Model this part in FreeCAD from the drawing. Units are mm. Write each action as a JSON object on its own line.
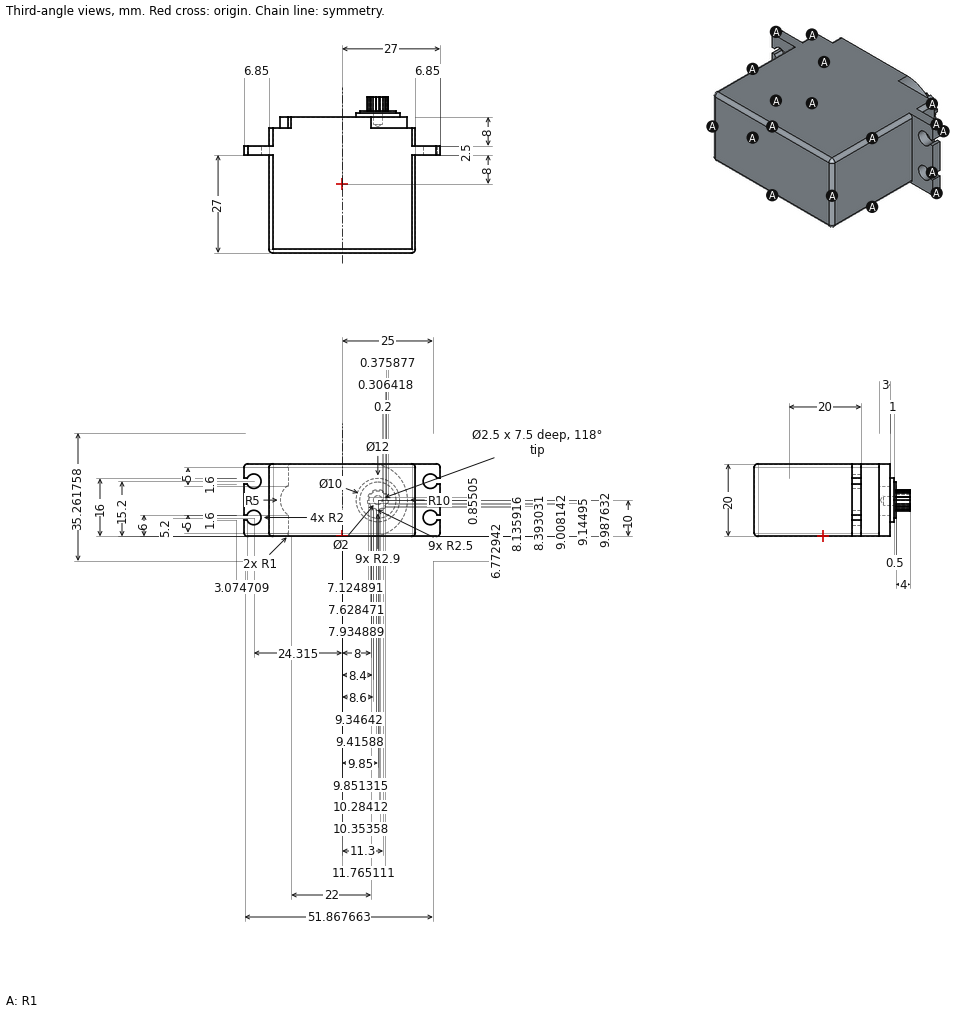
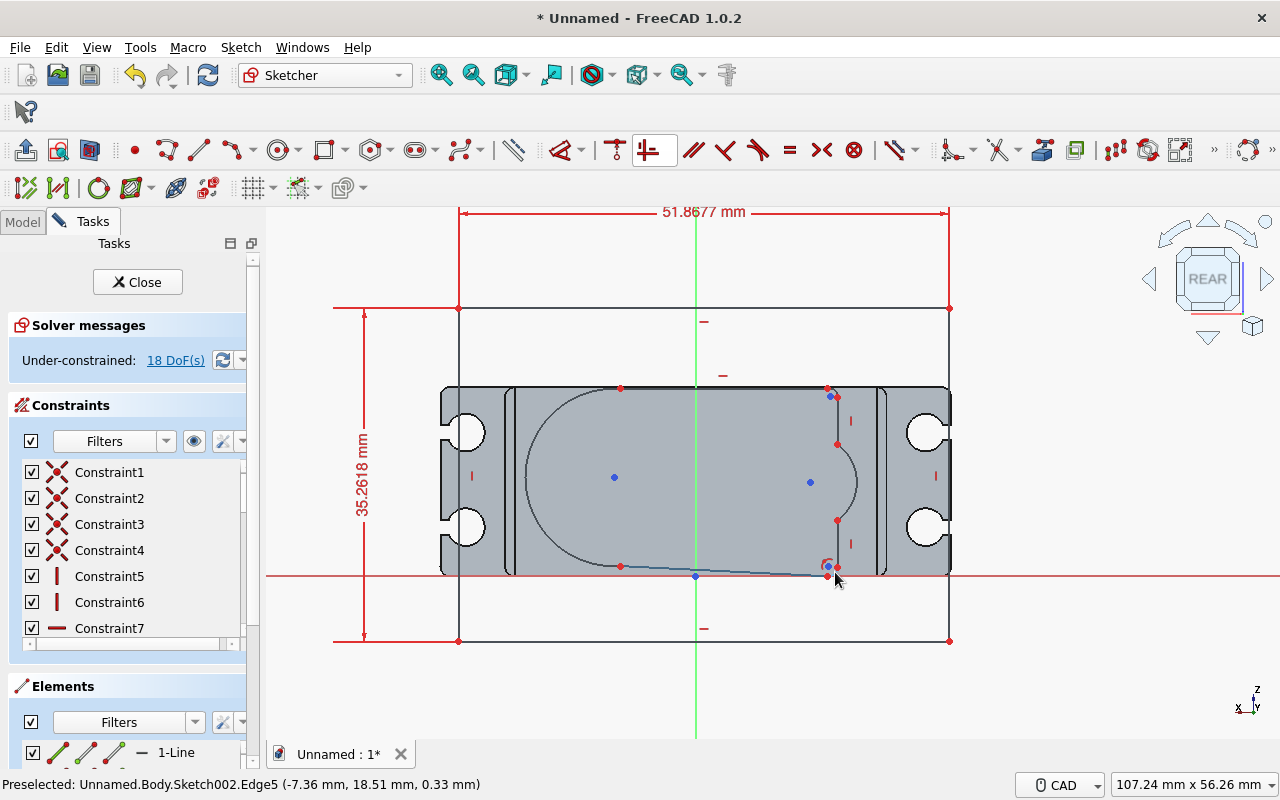
{"action": "left_click", "coordinate": [544, 423]}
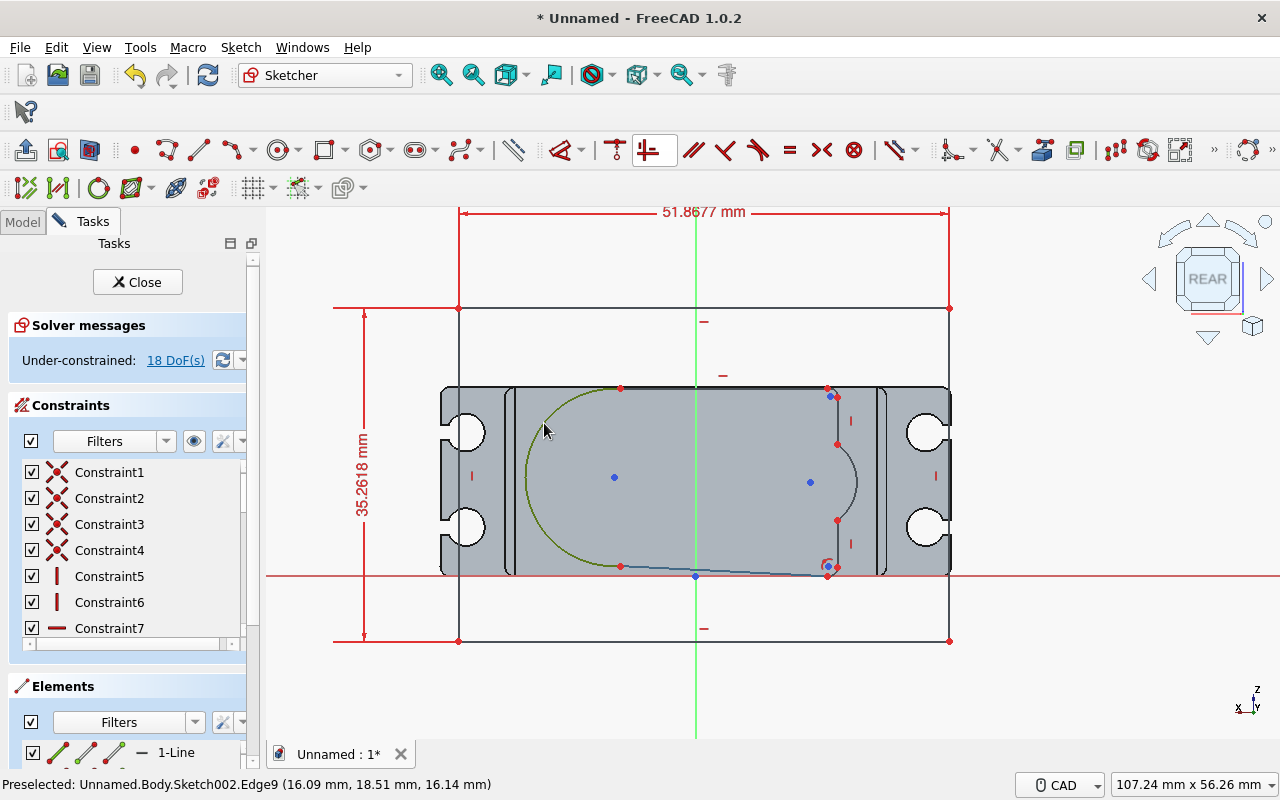
{"action": "left_click", "coordinate": [758, 150]}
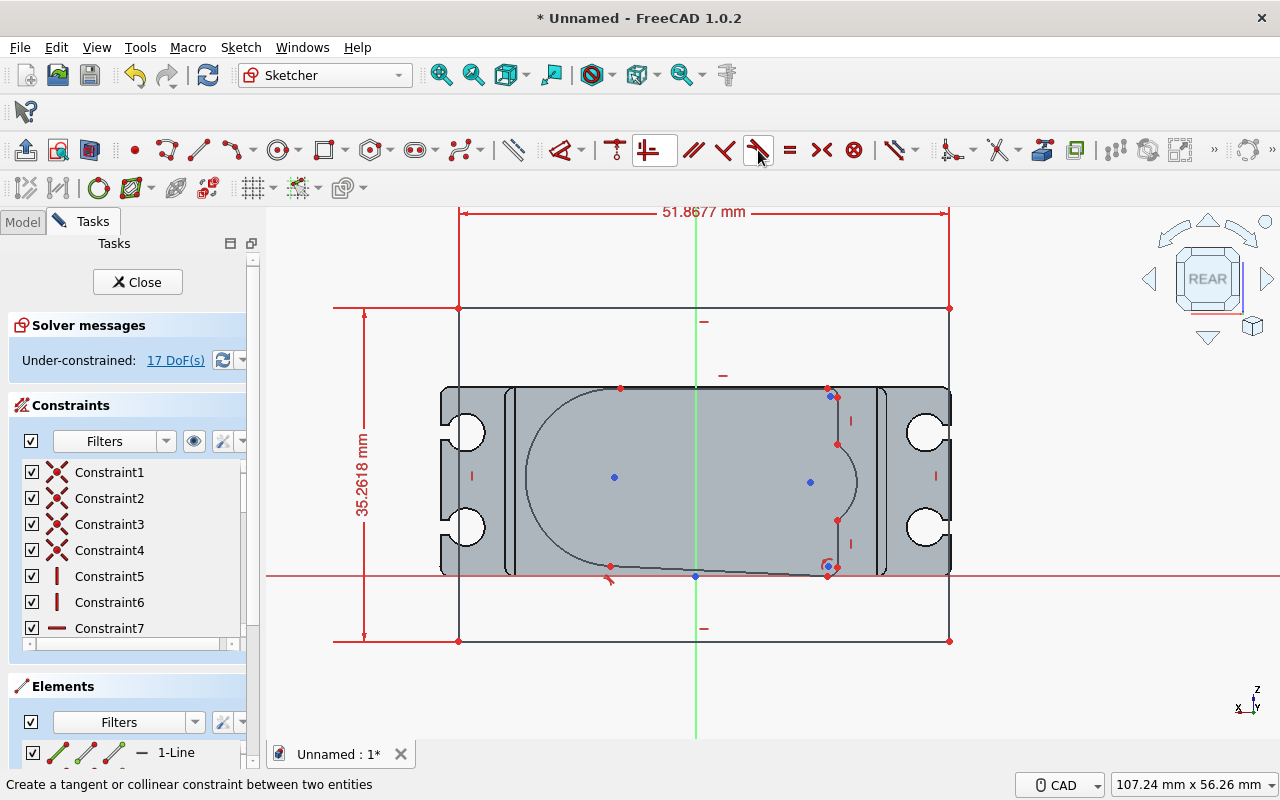
{"action": "left_click", "coordinate": [762, 573]}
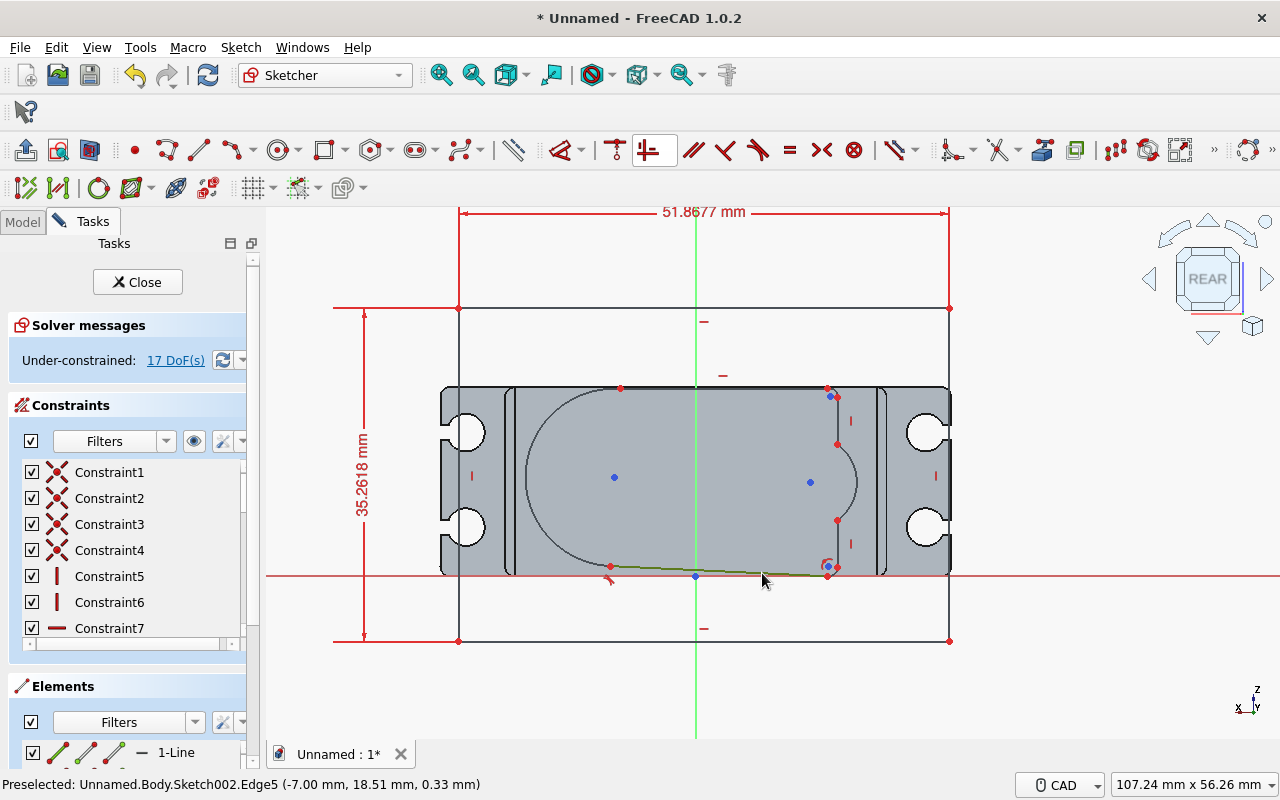
{"action": "scroll", "coordinate": [835, 574], "scroll_direction": "up", "scroll_amount": 4}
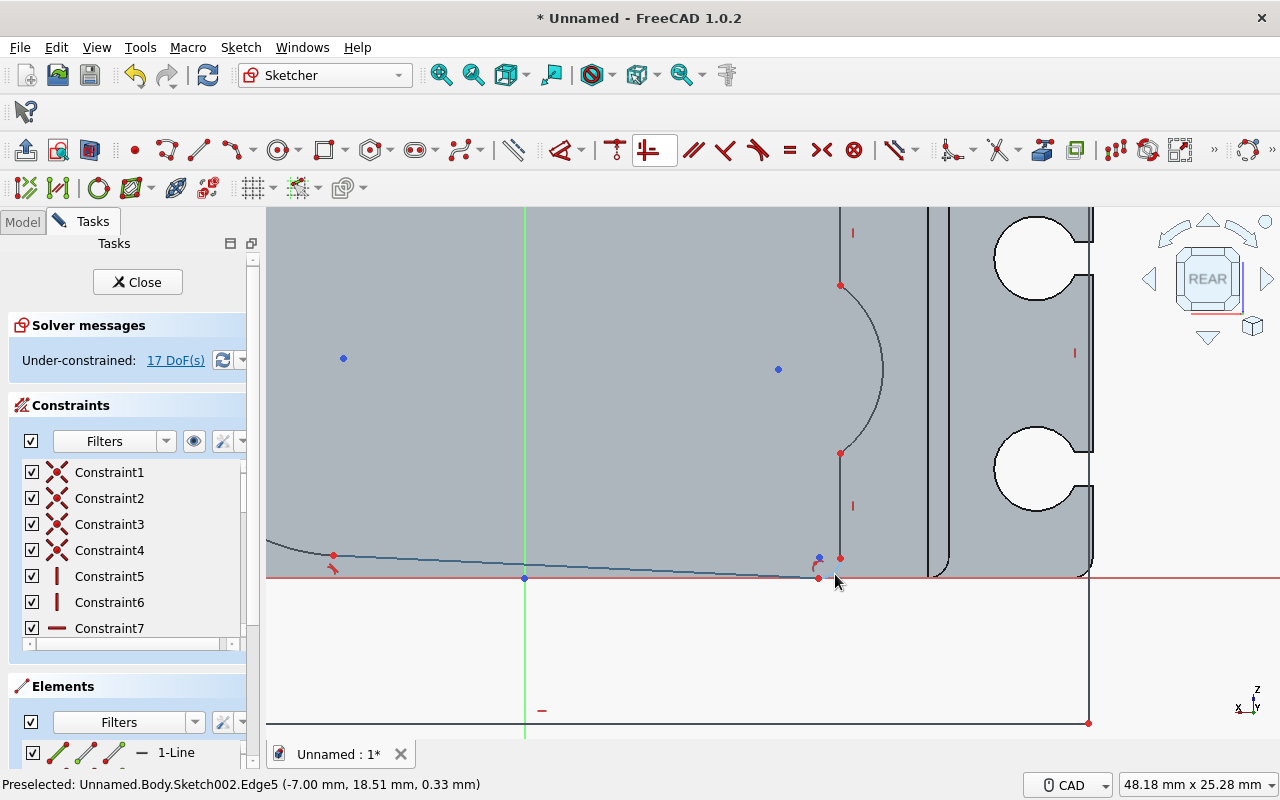
{"action": "left_click", "coordinate": [833, 573]}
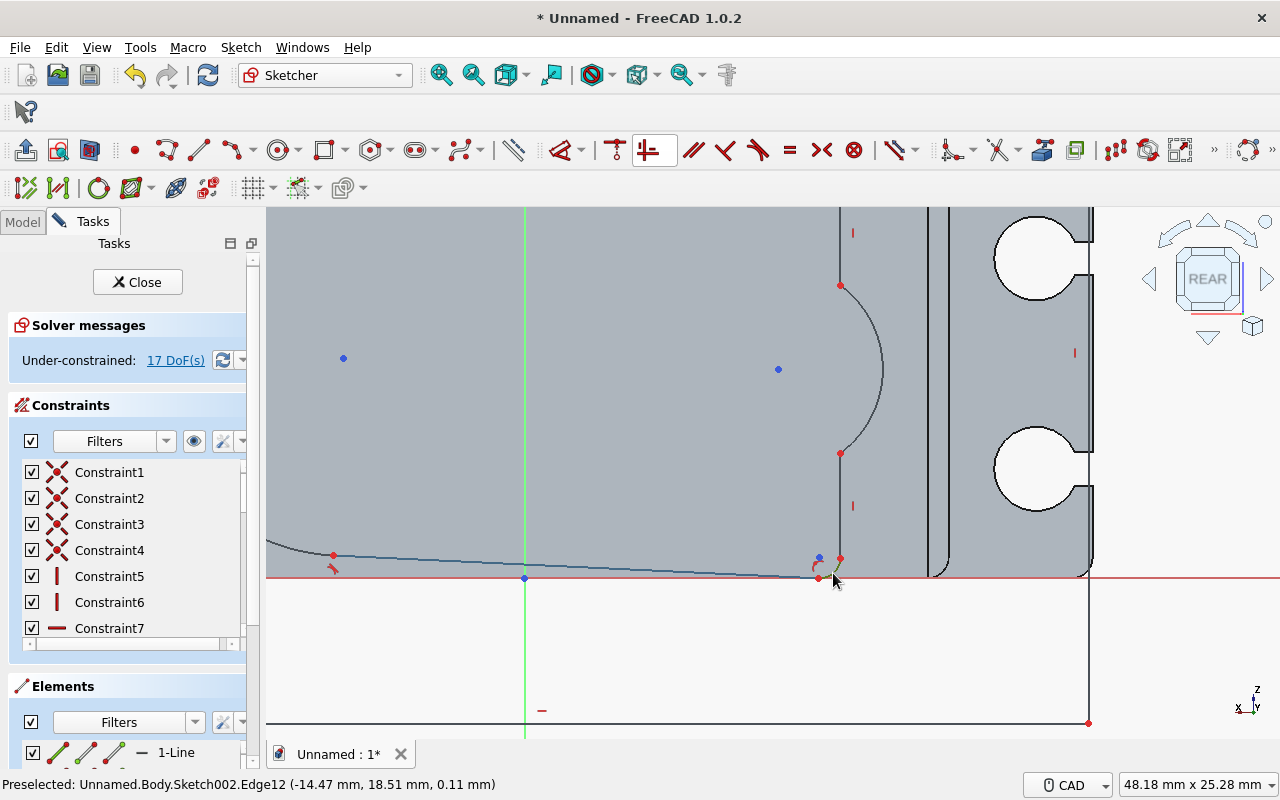
{"action": "left_click", "coordinate": [758, 150]}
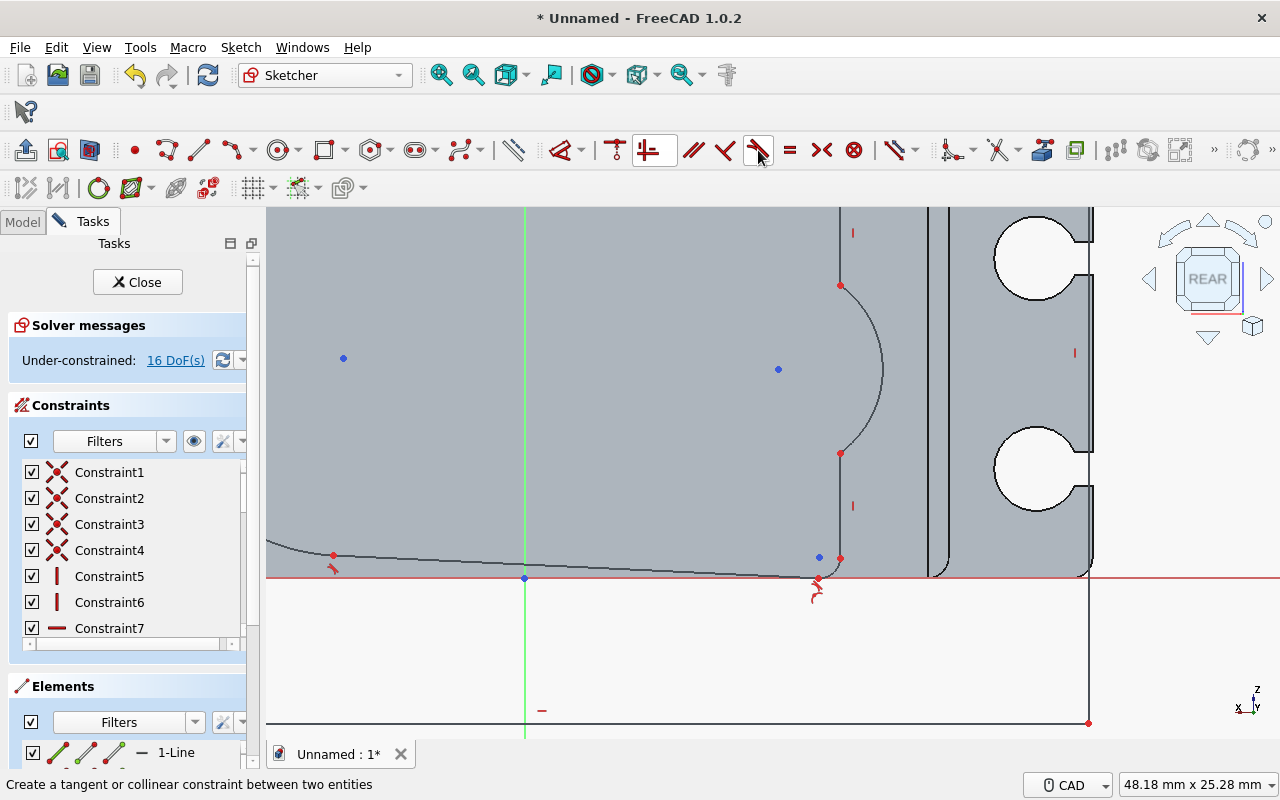
{"action": "scroll", "coordinate": [835, 573], "scroll_direction": "down", "scroll_amount": 4}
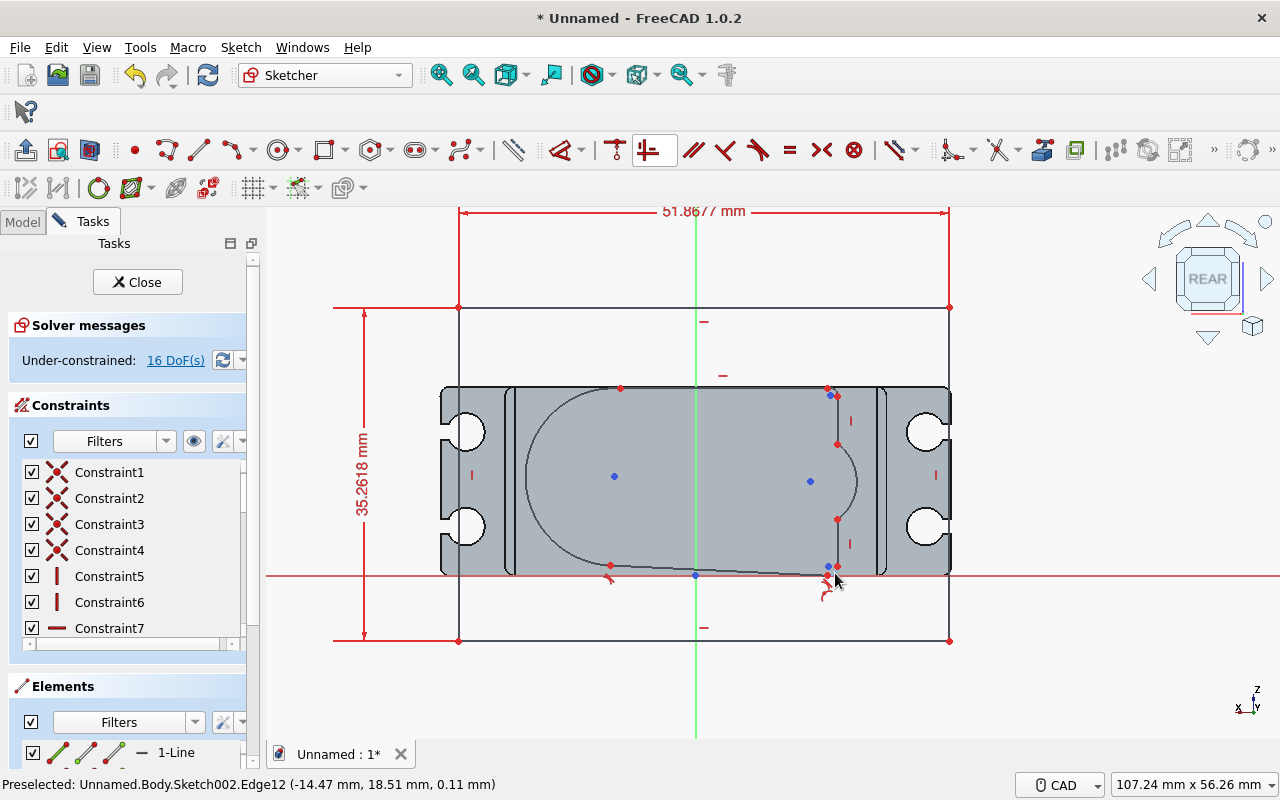
{"action": "left_click", "coordinate": [682, 388]}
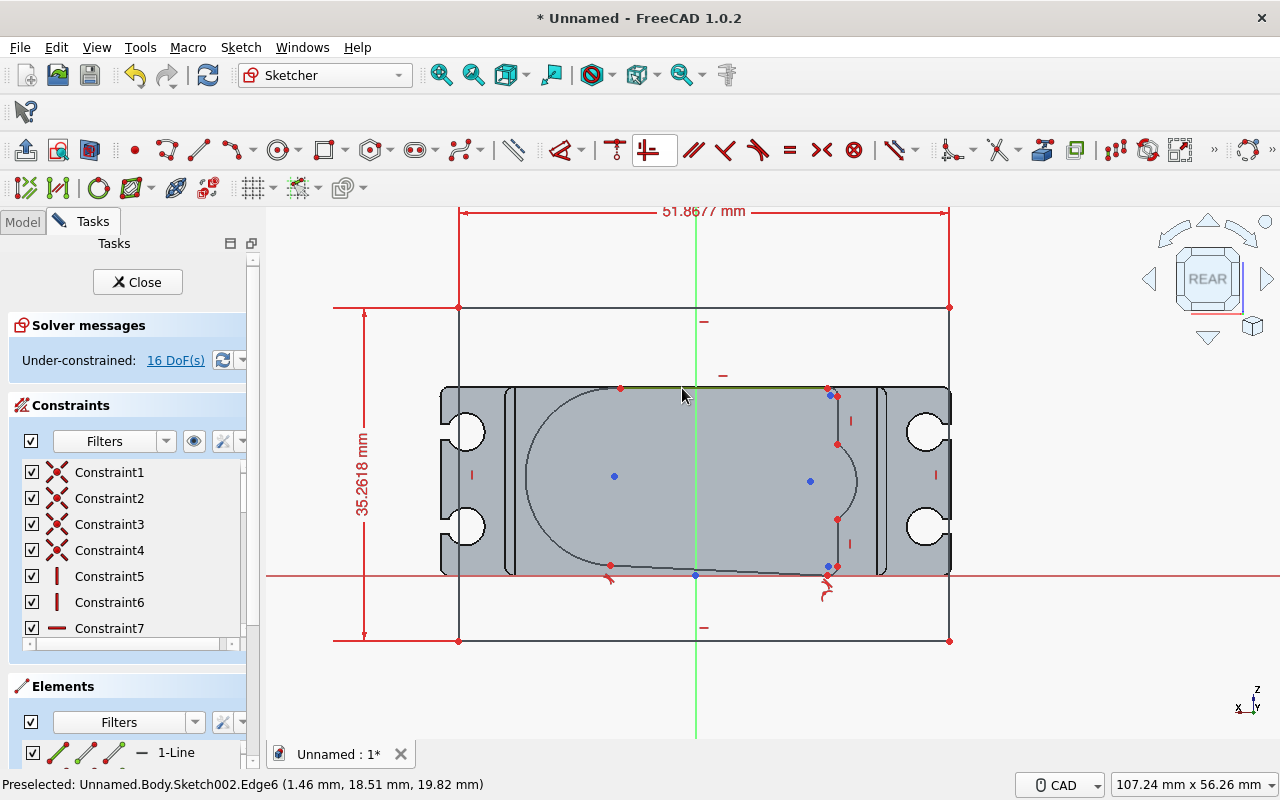
{"action": "left_click", "coordinate": [546, 421]}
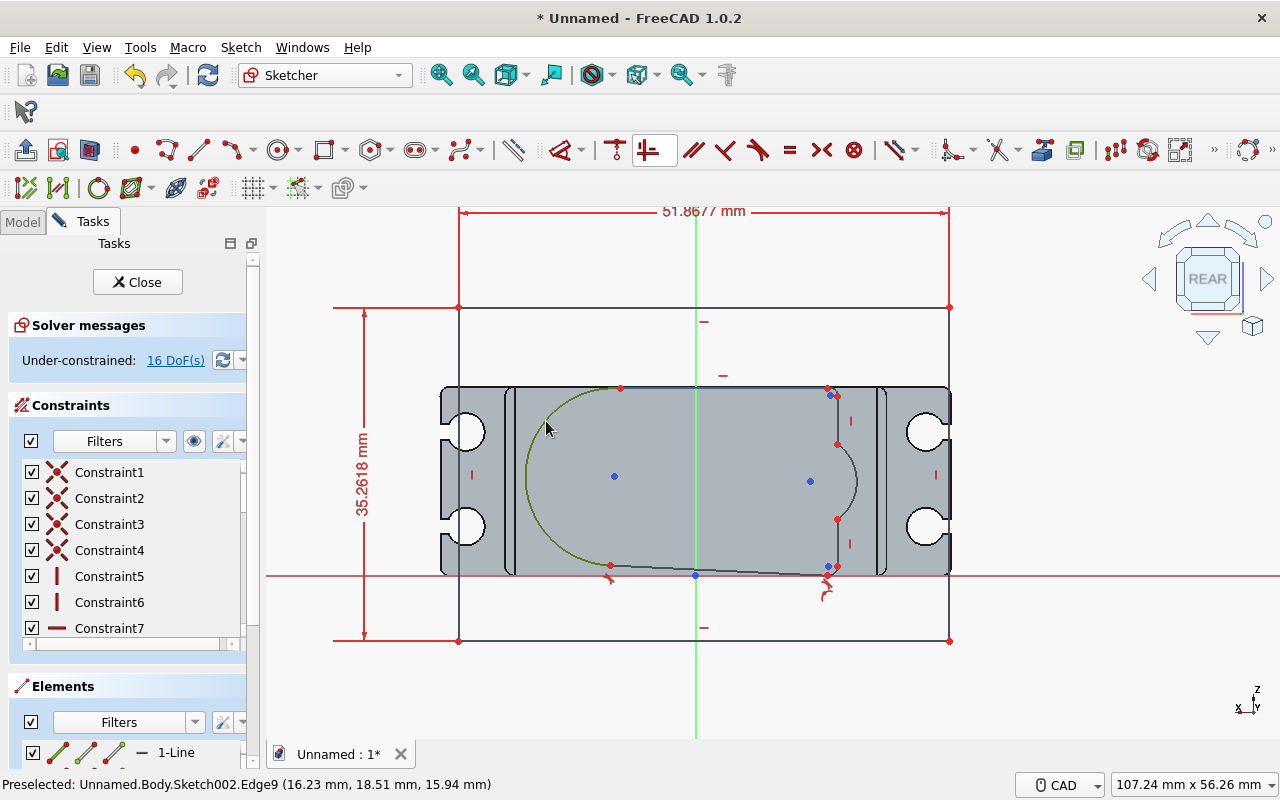
{"action": "left_click", "coordinate": [758, 150]}